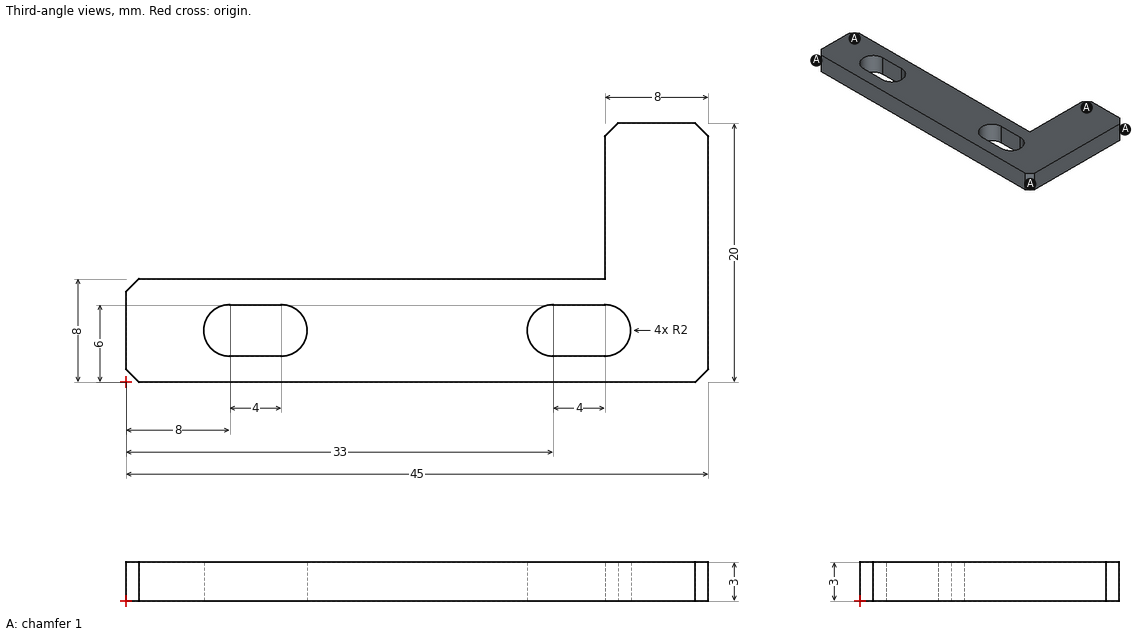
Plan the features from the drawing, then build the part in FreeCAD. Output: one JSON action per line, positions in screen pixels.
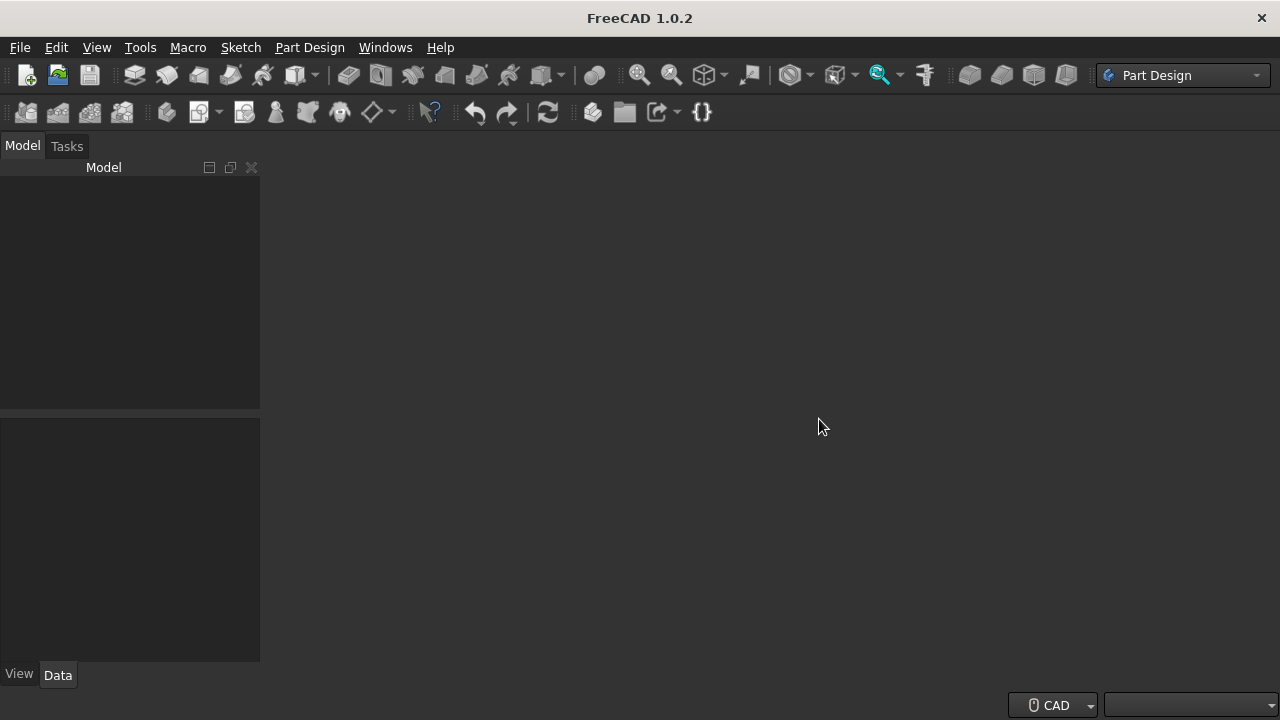
{"action": "left_click", "coordinate": [26, 76]}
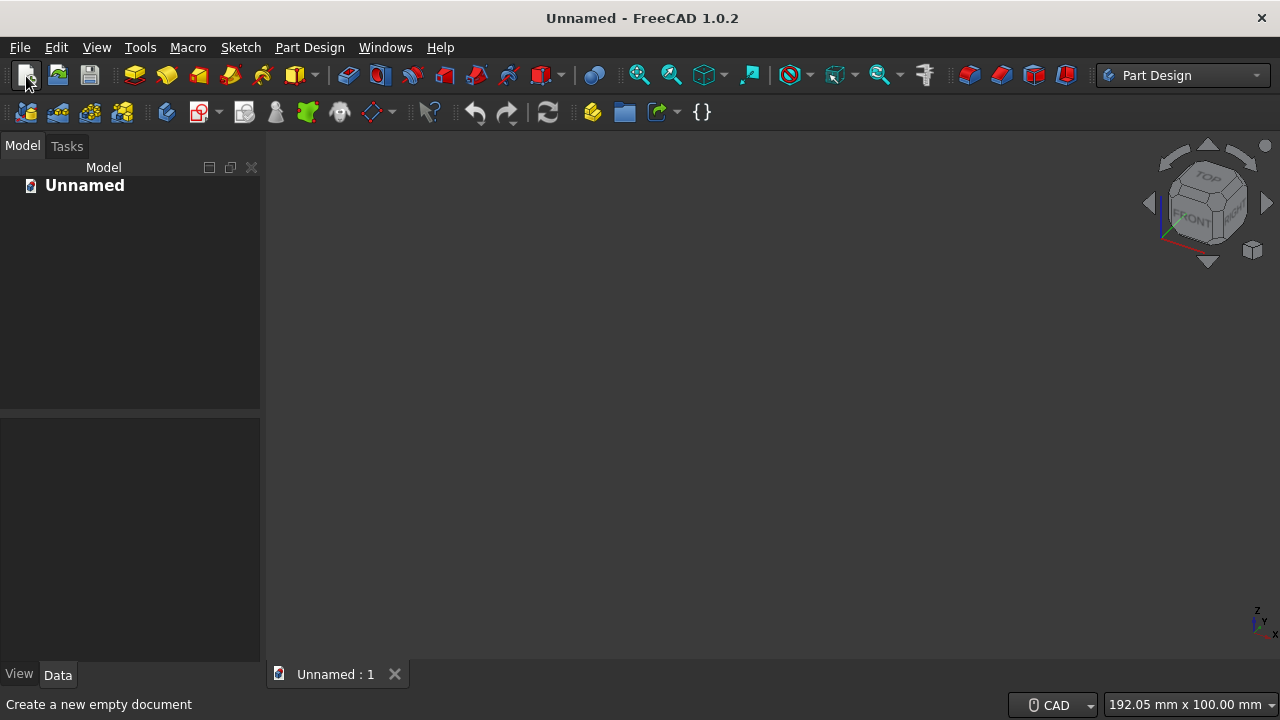
{"action": "left_click", "coordinate": [200, 112]}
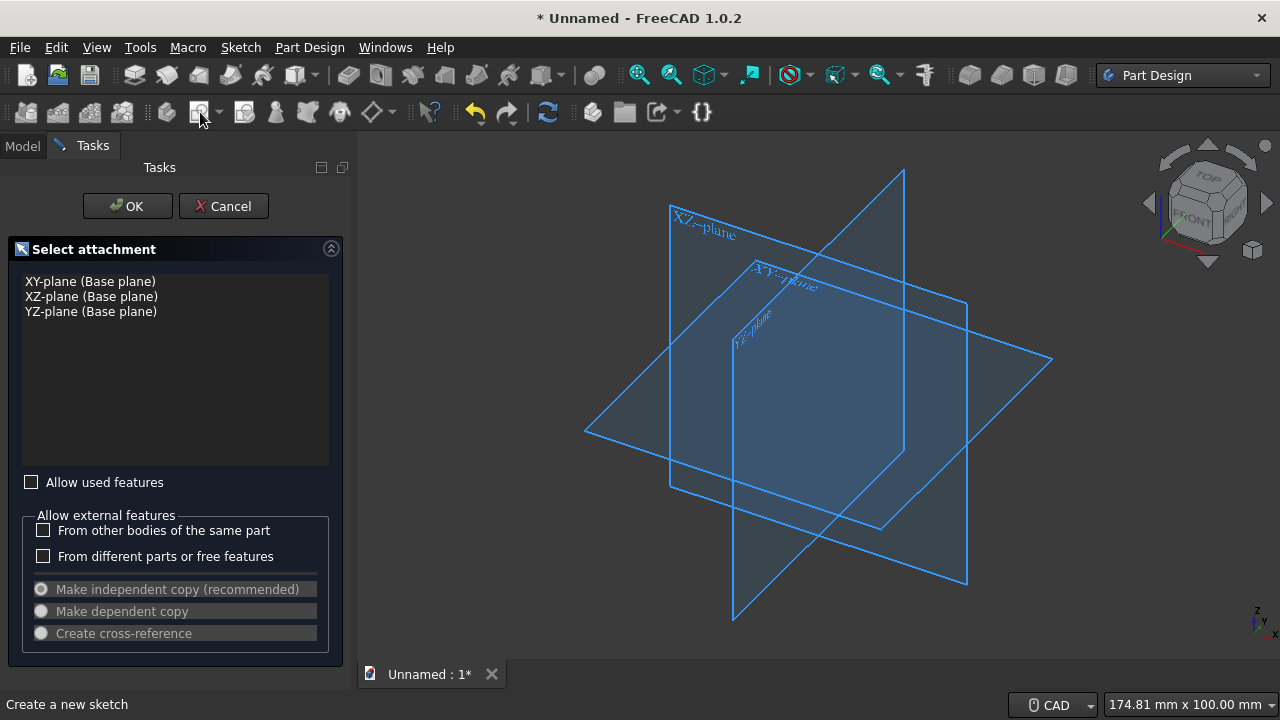
{"action": "left_click", "coordinate": [82, 282]}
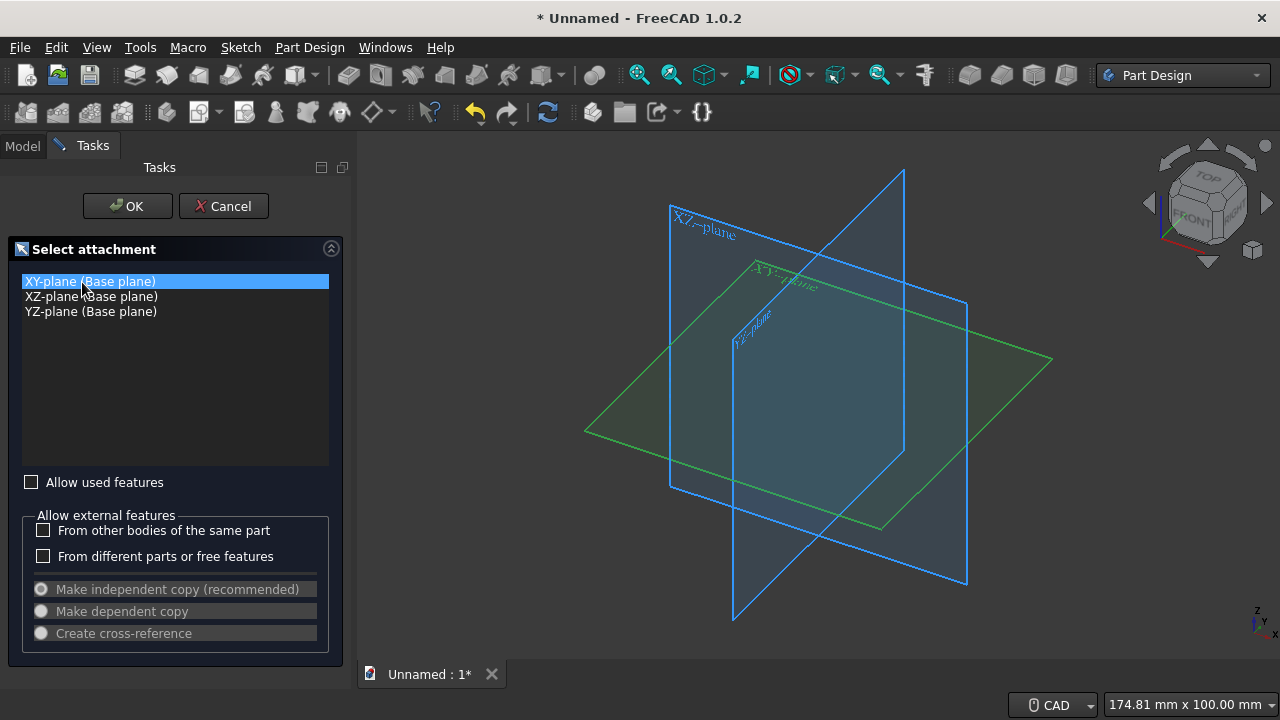
{"action": "left_click", "coordinate": [128, 206]}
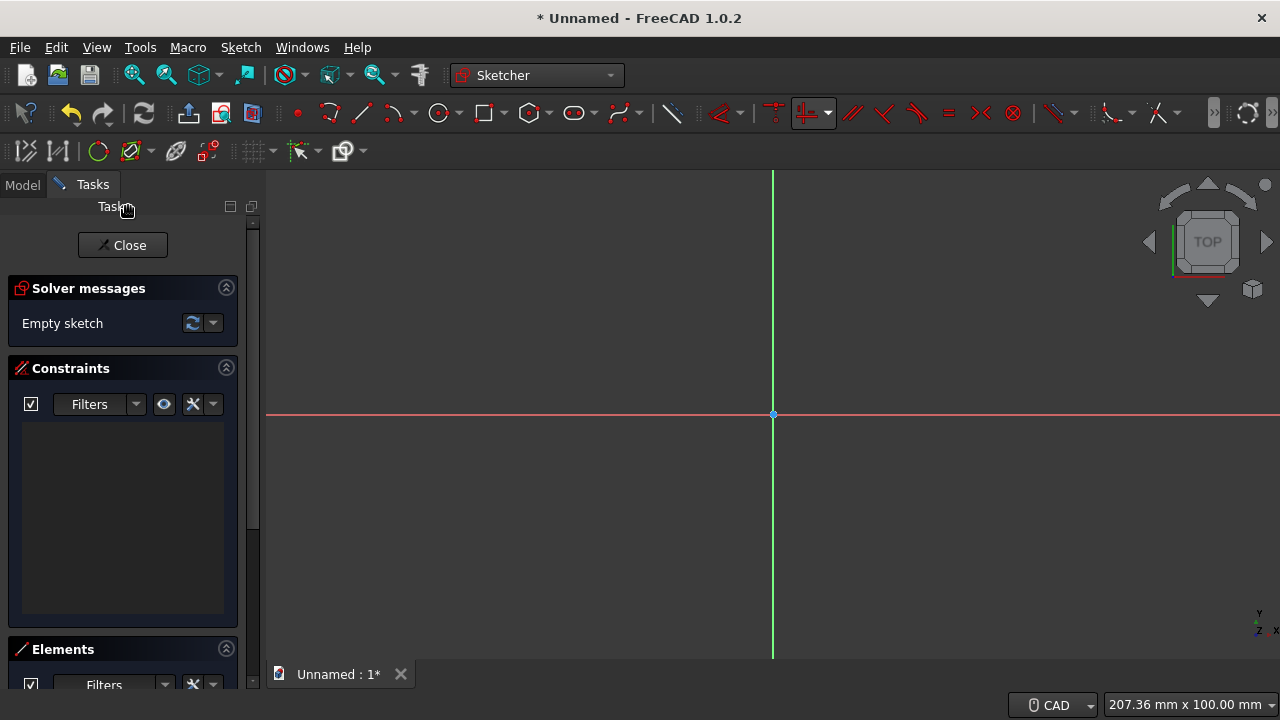
{"action": "scroll", "coordinate": [987, 337], "scroll_direction": "up", "scroll_amount": 5}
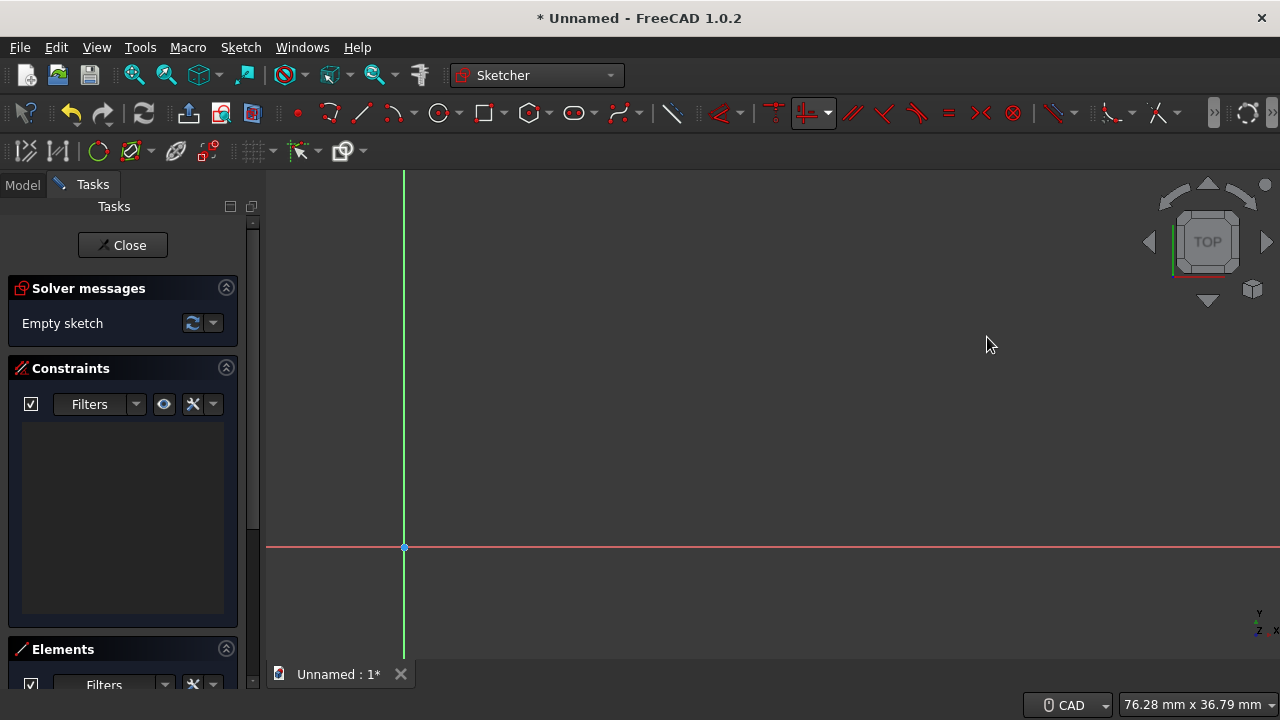
{"action": "left_click", "coordinate": [330, 114]}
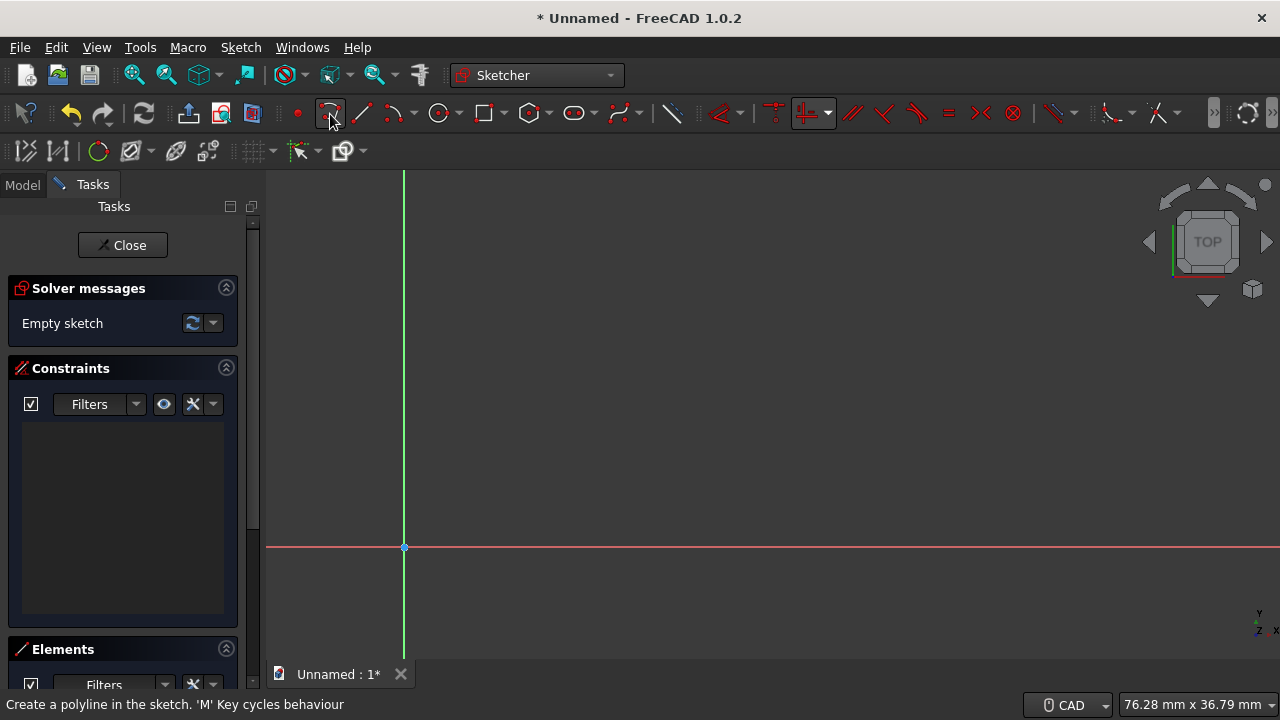
{"action": "left_click", "coordinate": [404, 547]}
{"action": "left_click", "coordinate": [1002, 538]}
{"action": "left_click", "coordinate": [1002, 281]}
{"action": "left_click", "coordinate": [896, 281]}
{"action": "left_click", "coordinate": [896, 441]}
{"action": "left_click", "coordinate": [413, 441]}
{"action": "left_click", "coordinate": [404, 547]}
{"action": "key", "text": "Escape"}
{"action": "key", "text": "Escape"}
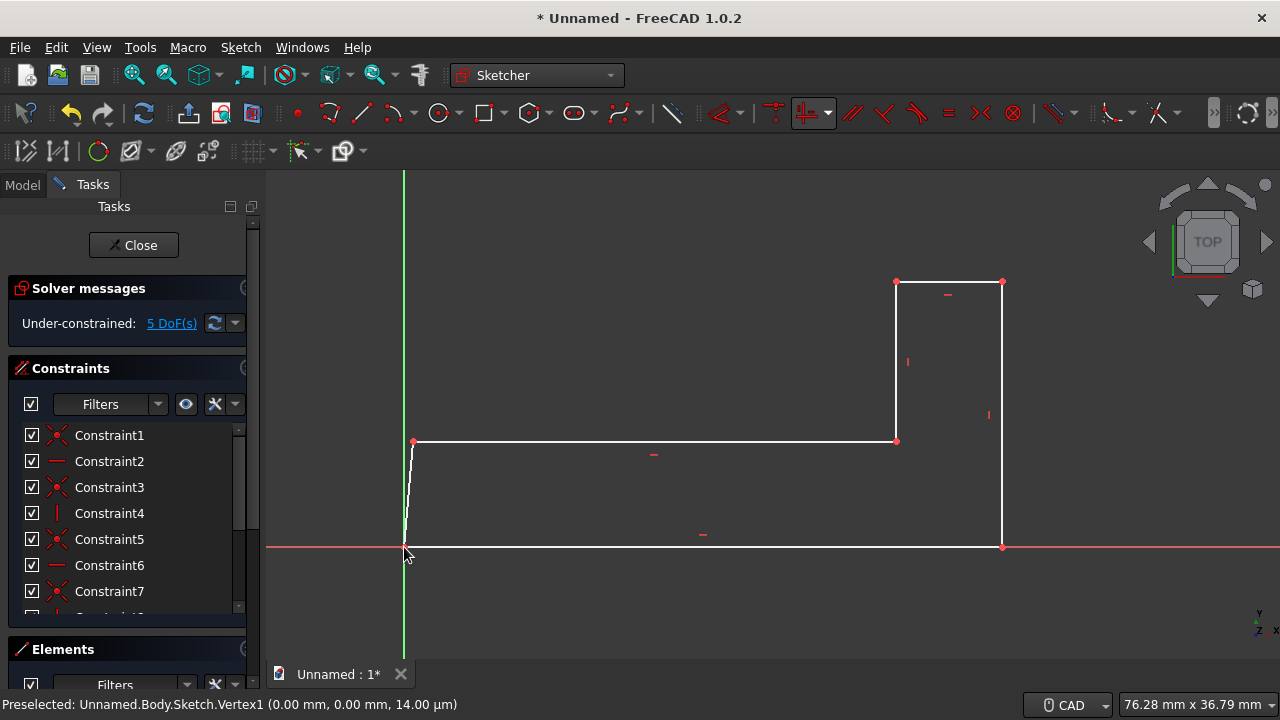
{"action": "left_click", "coordinate": [407, 516]}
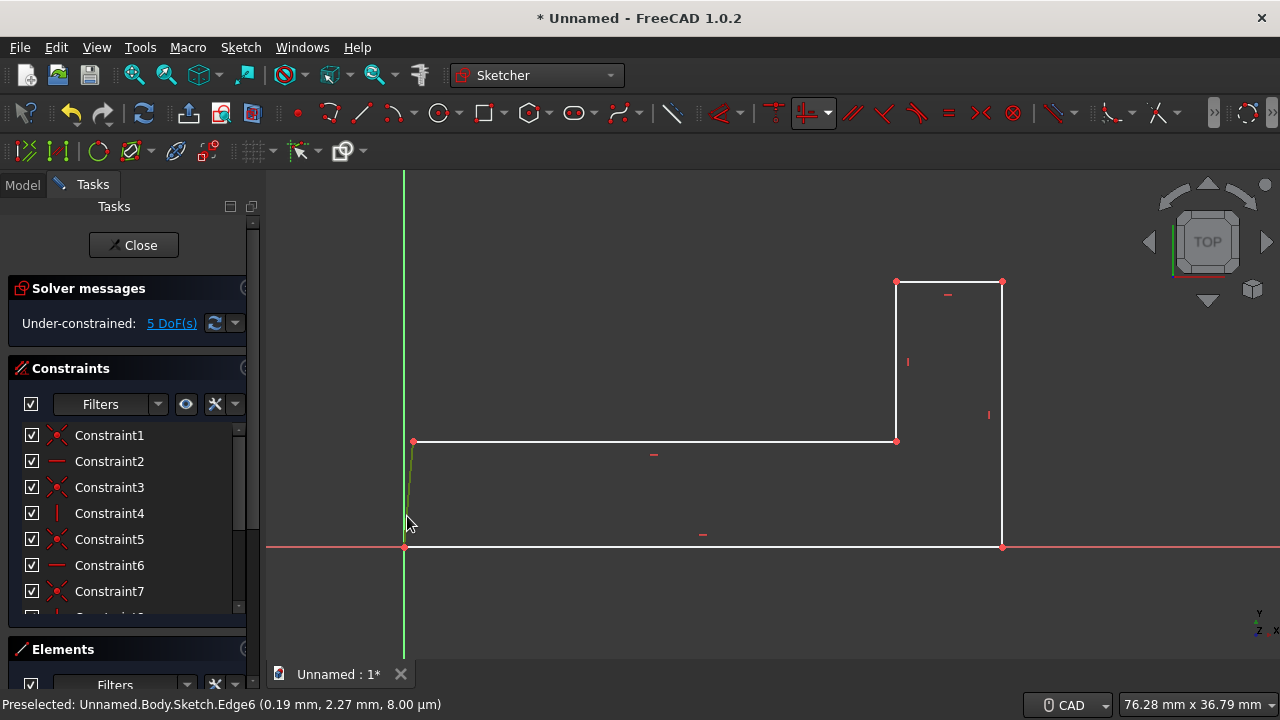
{"action": "left_click", "coordinate": [830, 114]}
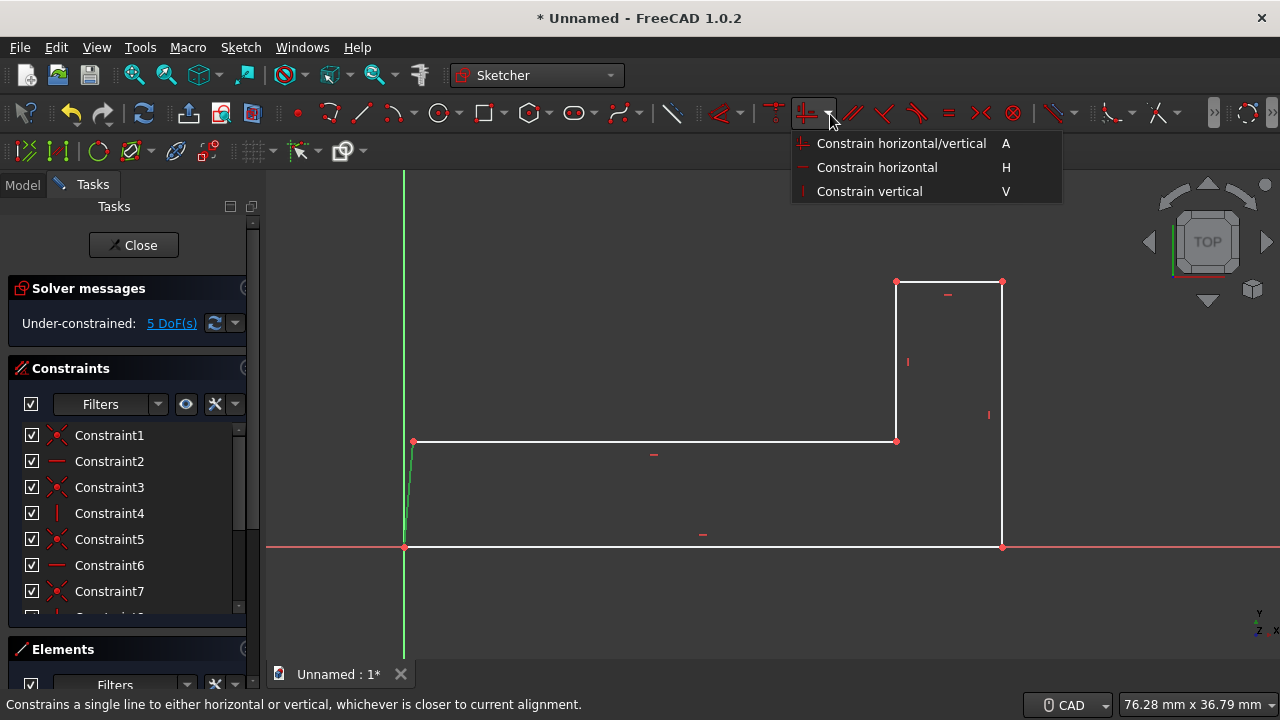
{"action": "left_click", "coordinate": [927, 191]}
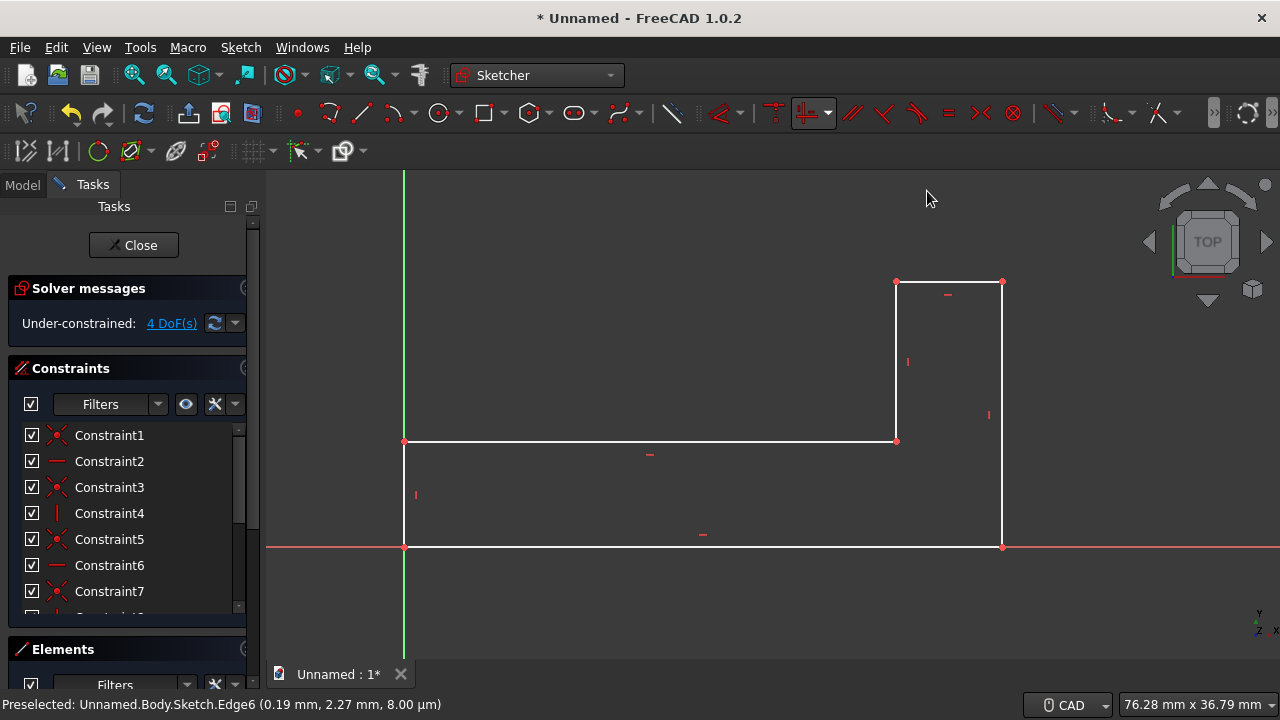
{"action": "left_click", "coordinate": [720, 114]}